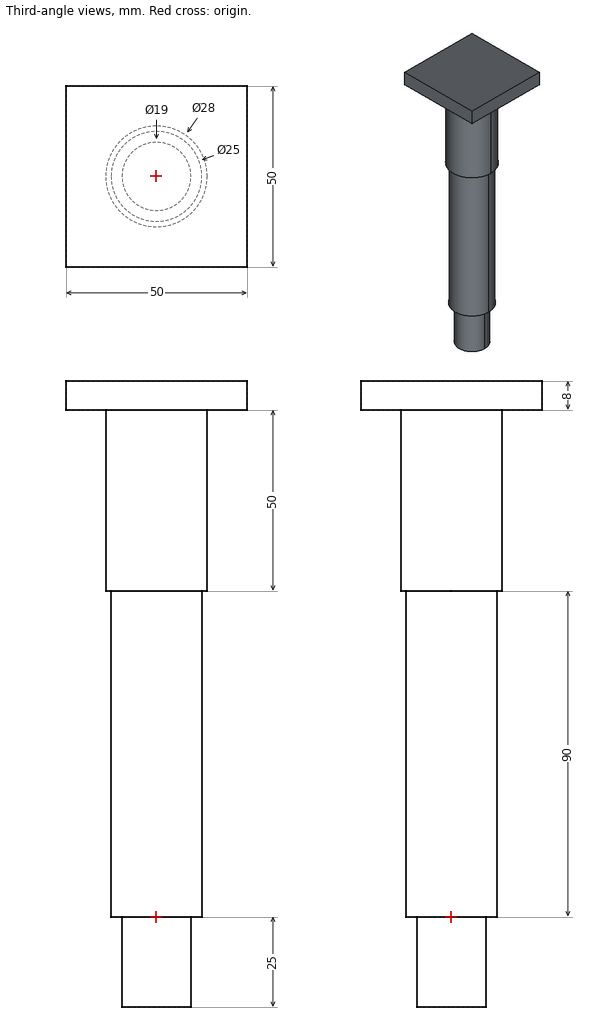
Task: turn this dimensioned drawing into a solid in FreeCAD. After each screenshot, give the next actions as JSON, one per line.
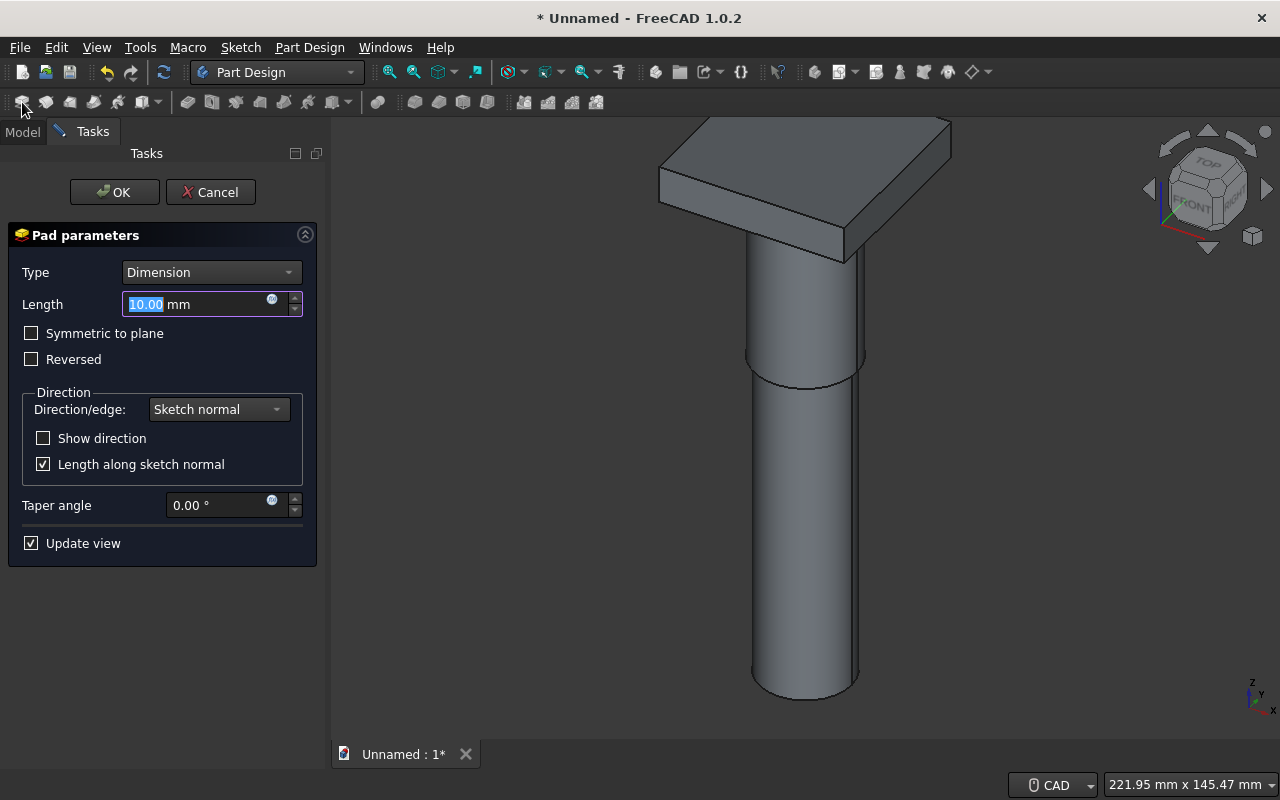
{"action": "type", "text": "8"}
{"action": "key", "text": "Tab"}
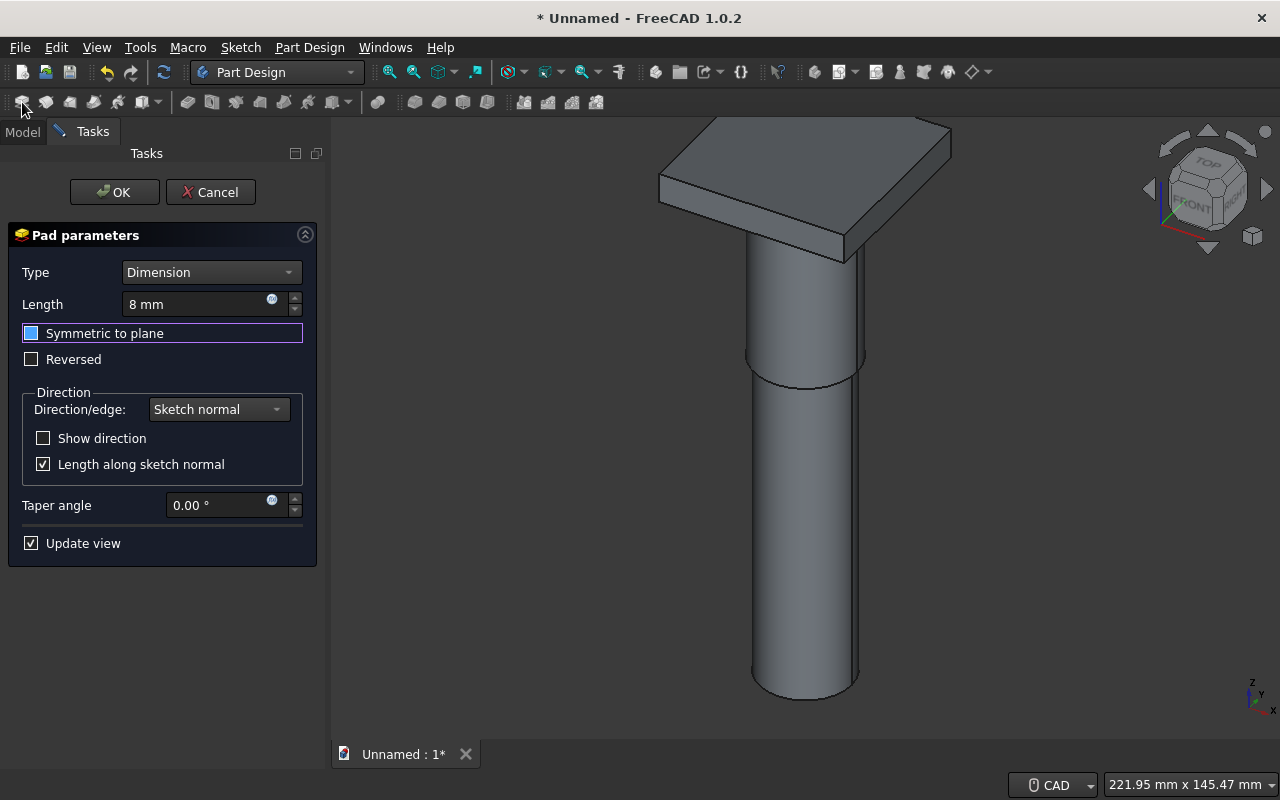
{"action": "left_click", "coordinate": [115, 192]}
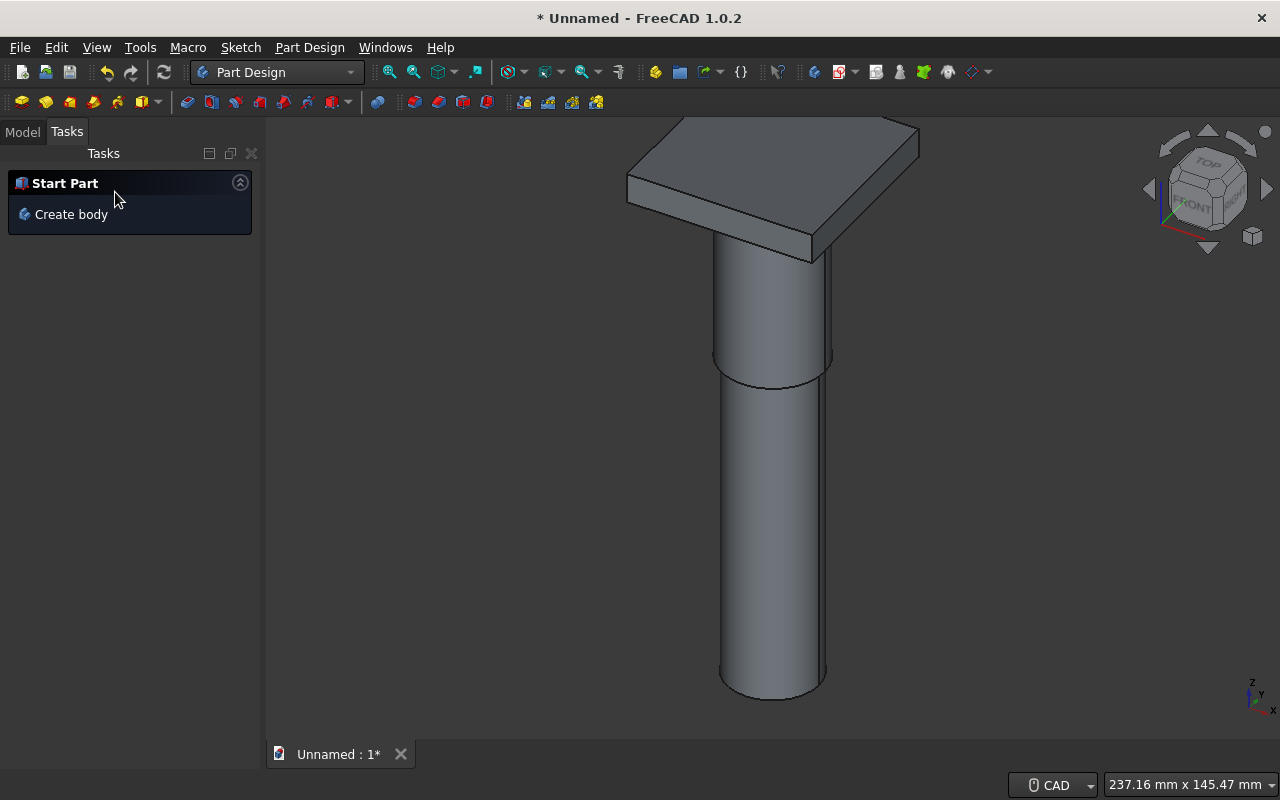
{"action": "key", "text": "v f"}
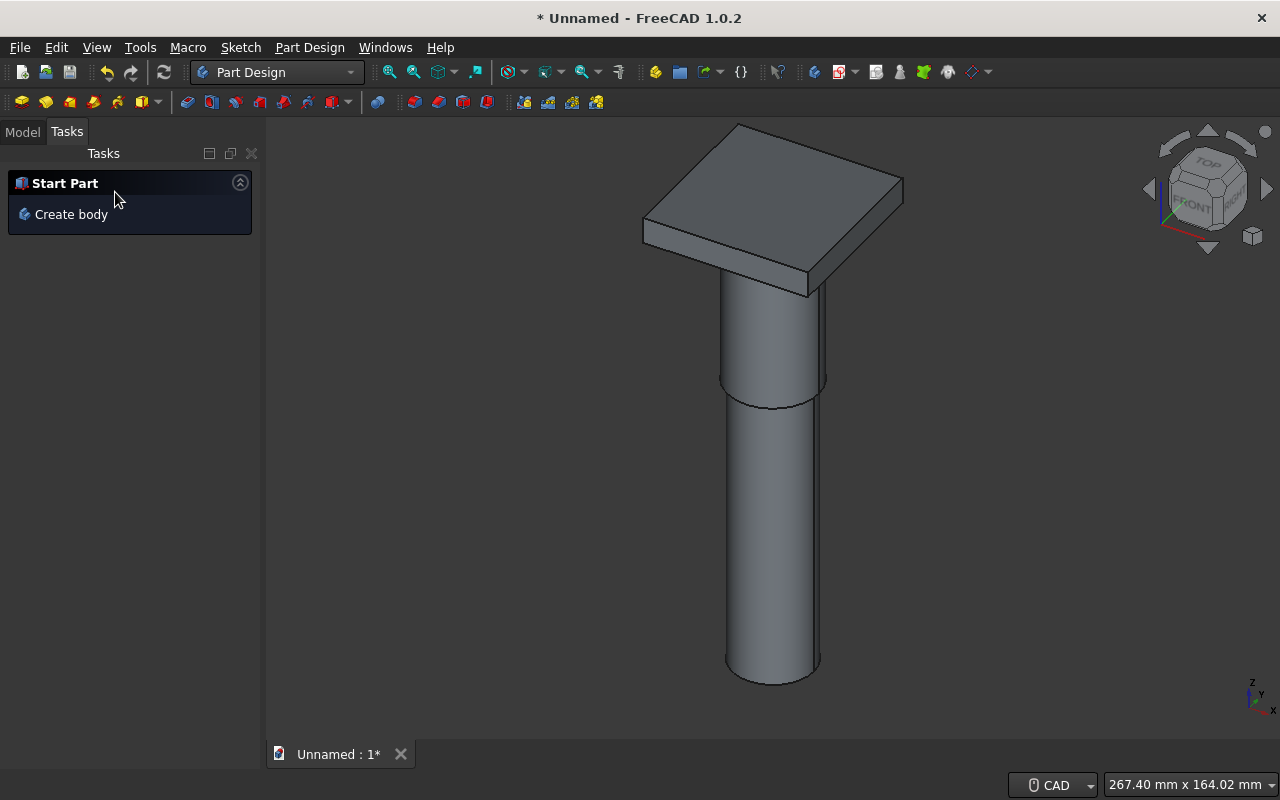
{"action": "left_click", "coordinate": [840, 72]}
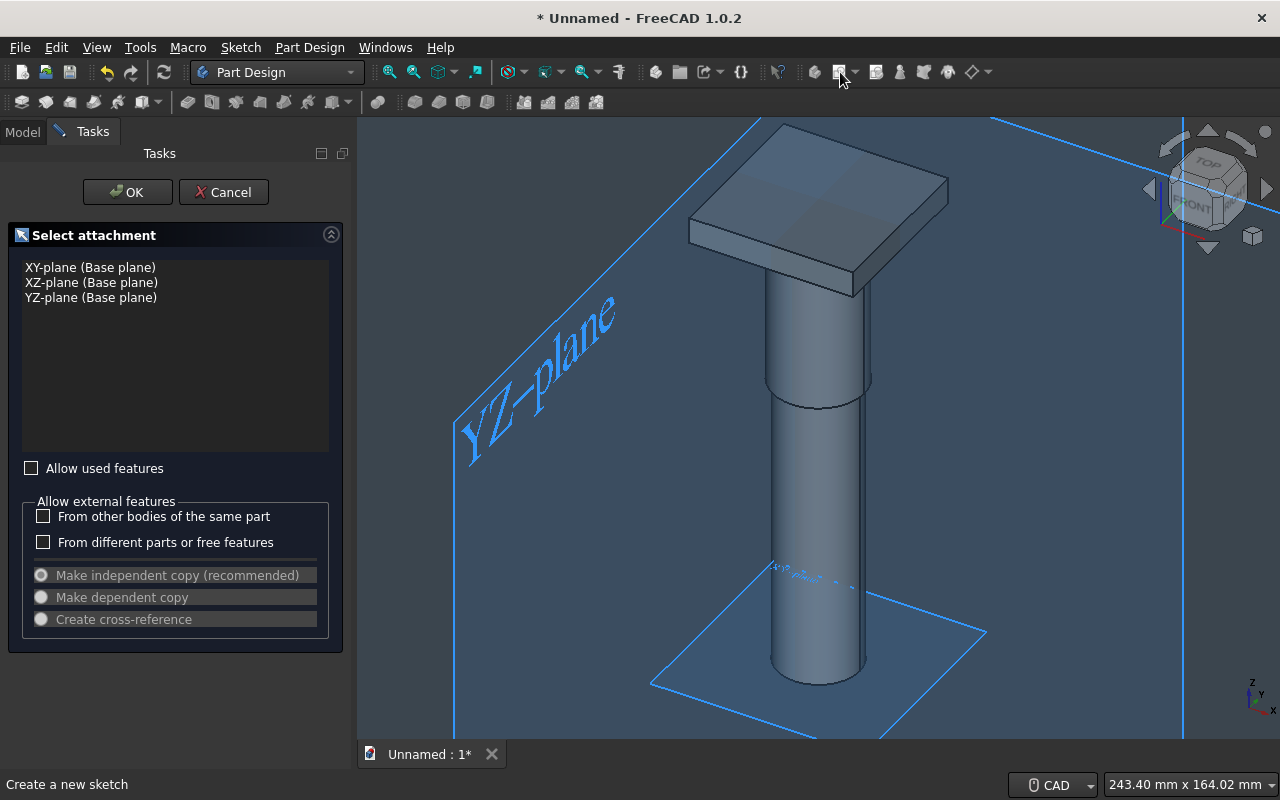
{"action": "left_click", "coordinate": [82, 268]}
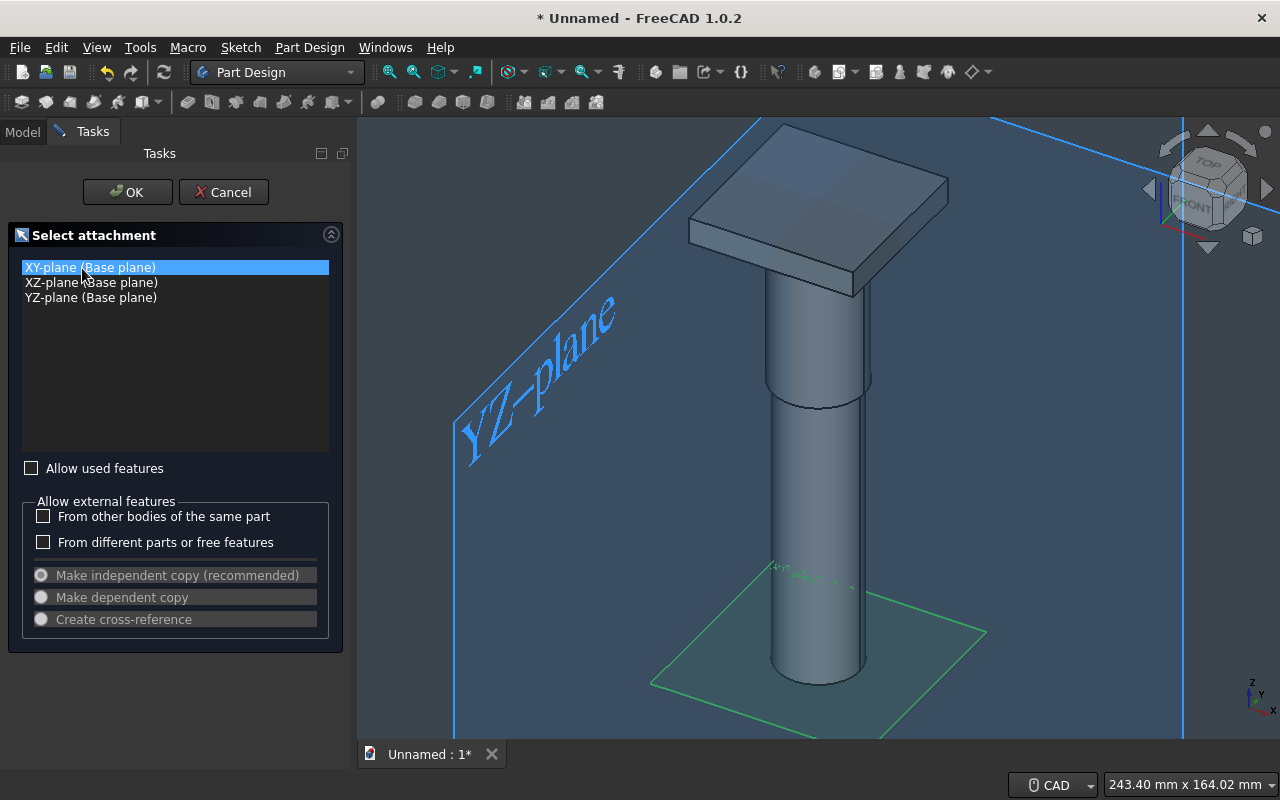
{"action": "left_click", "coordinate": [128, 192]}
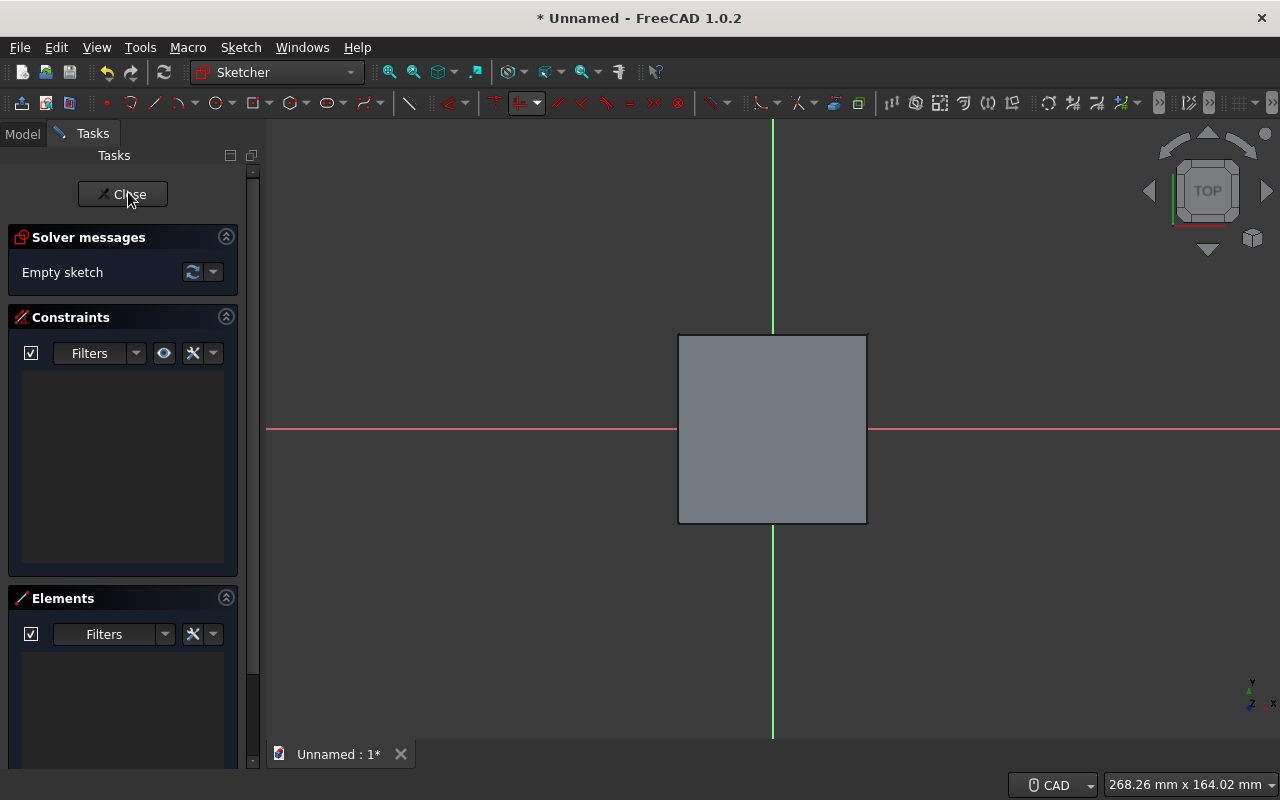
{"action": "left_click", "coordinate": [70, 104]}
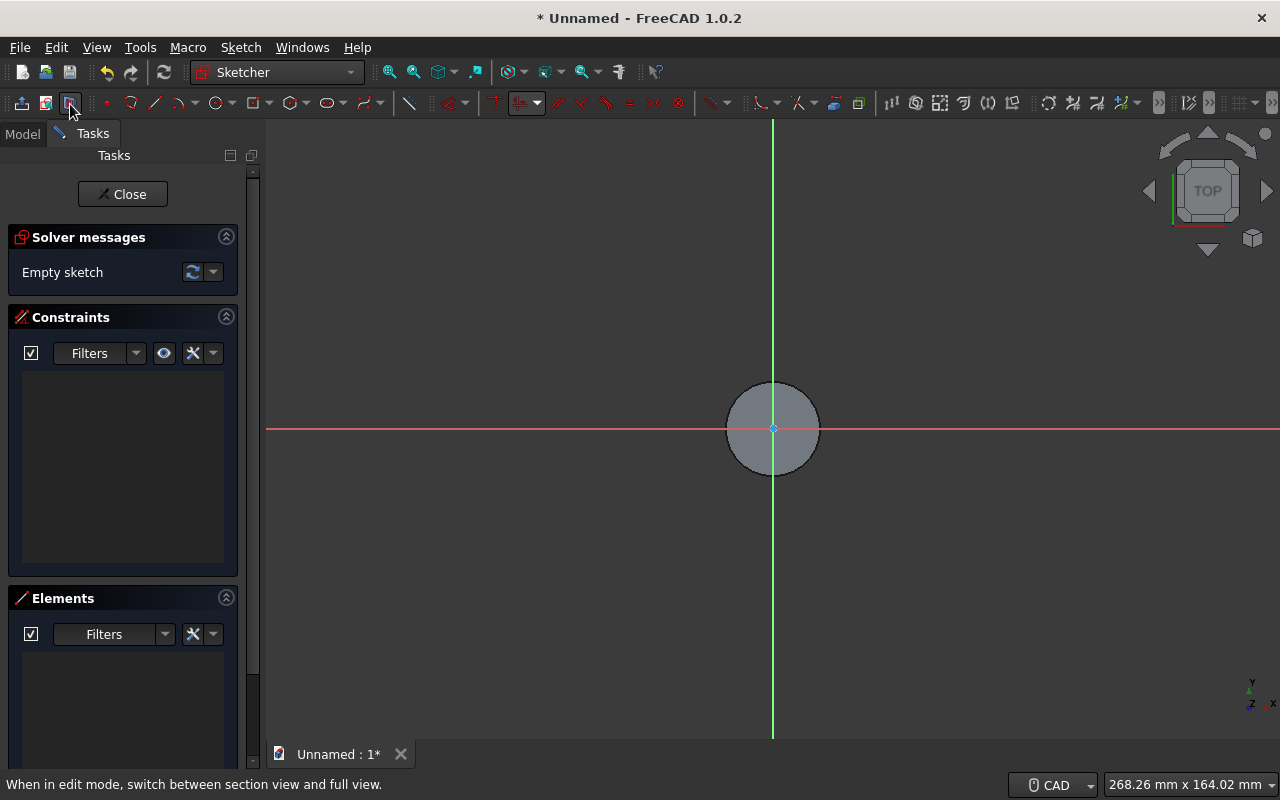
{"action": "scroll", "coordinate": [787, 429], "scroll_direction": "up", "scroll_amount": 9}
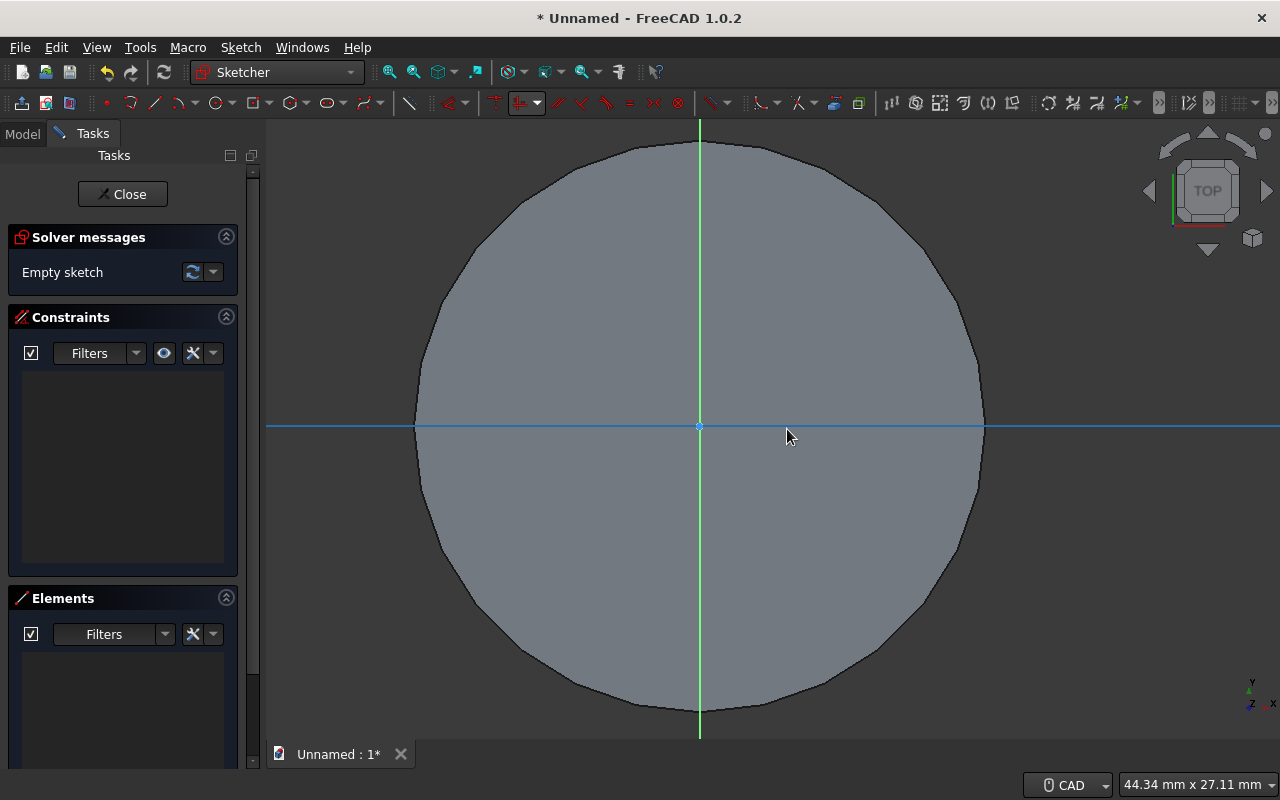
{"action": "key", "text": "g c"}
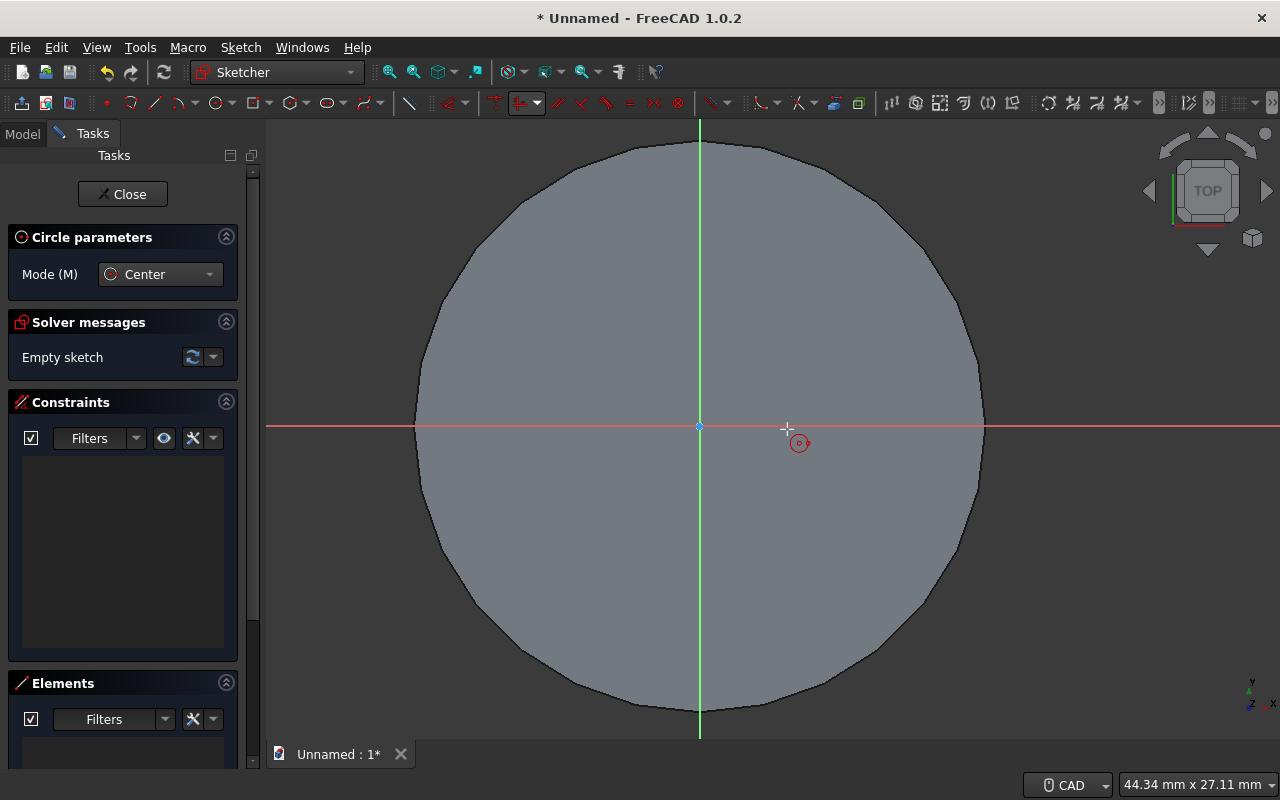
{"action": "left_click", "coordinate": [700, 426]}
{"action": "left_click", "coordinate": [853, 273]}
{"action": "key", "text": "Escape"}